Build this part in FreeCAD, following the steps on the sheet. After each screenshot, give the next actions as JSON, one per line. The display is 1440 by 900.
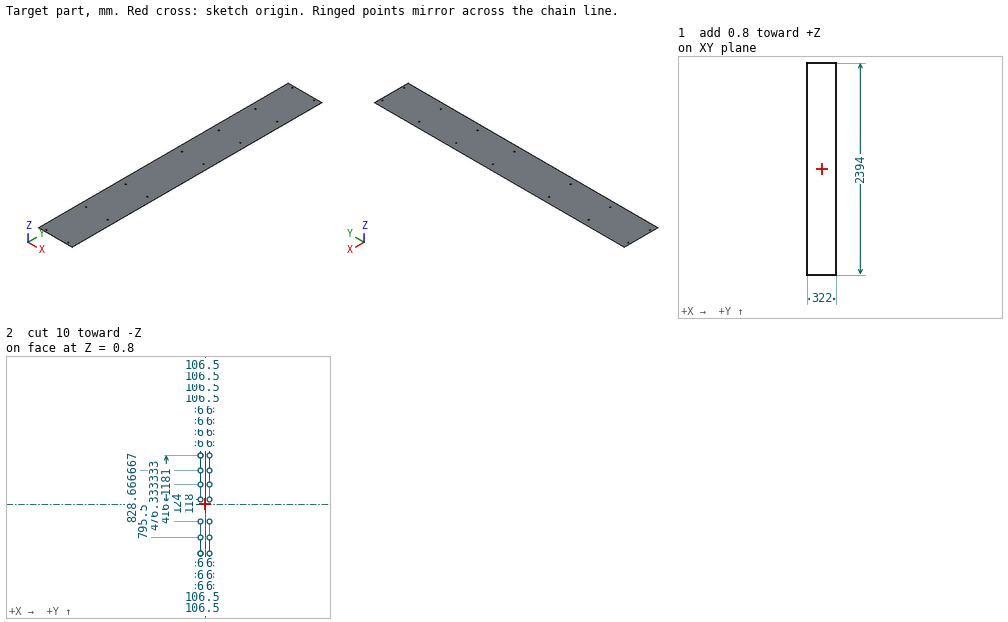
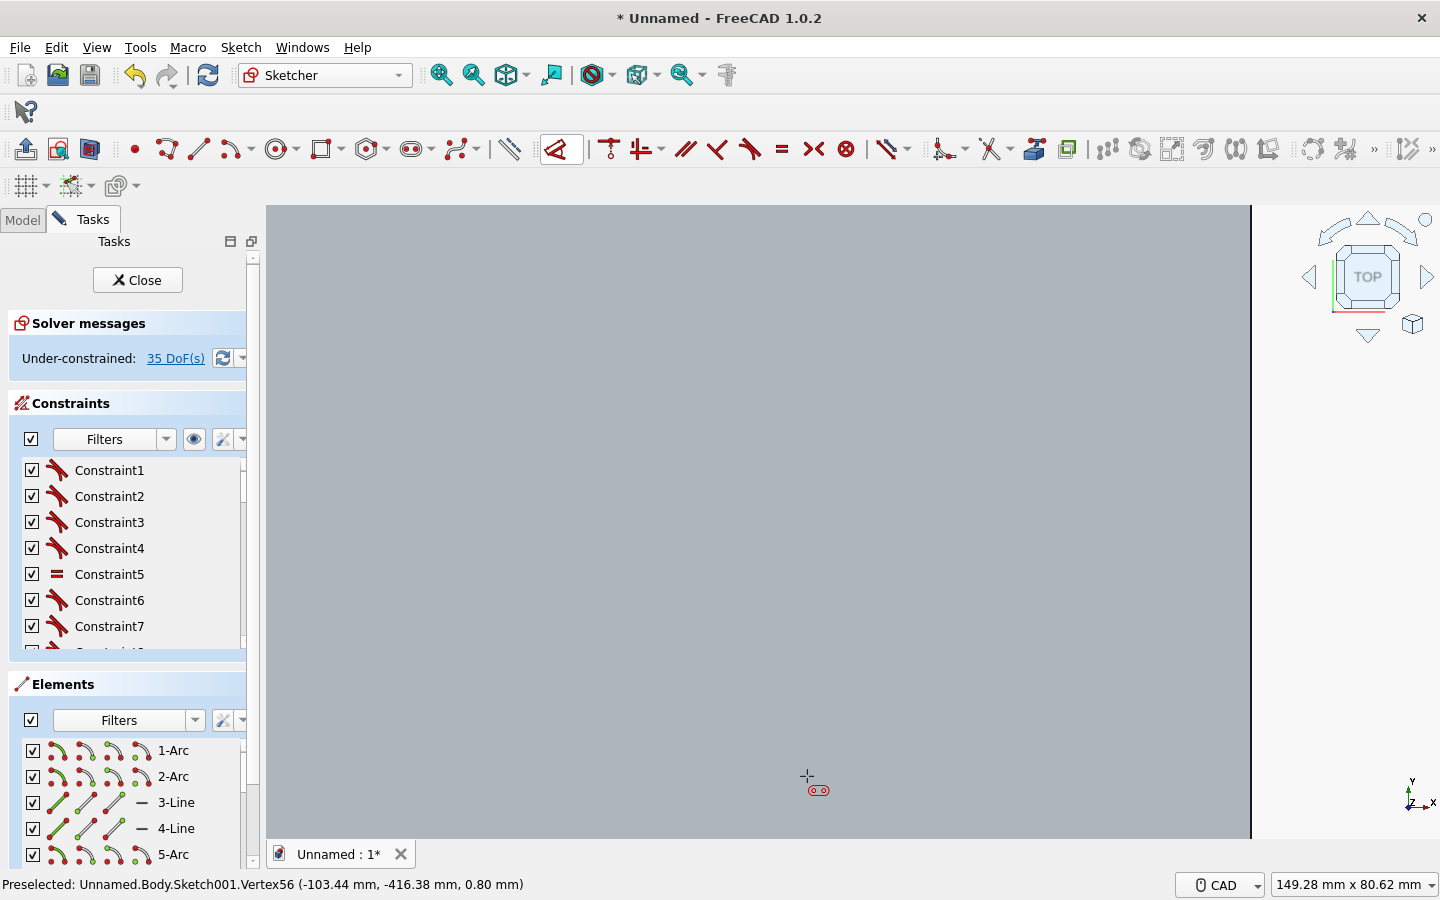
{"action": "scroll", "coordinate": [807, 776], "scroll_direction": "down", "scroll_amount": 18}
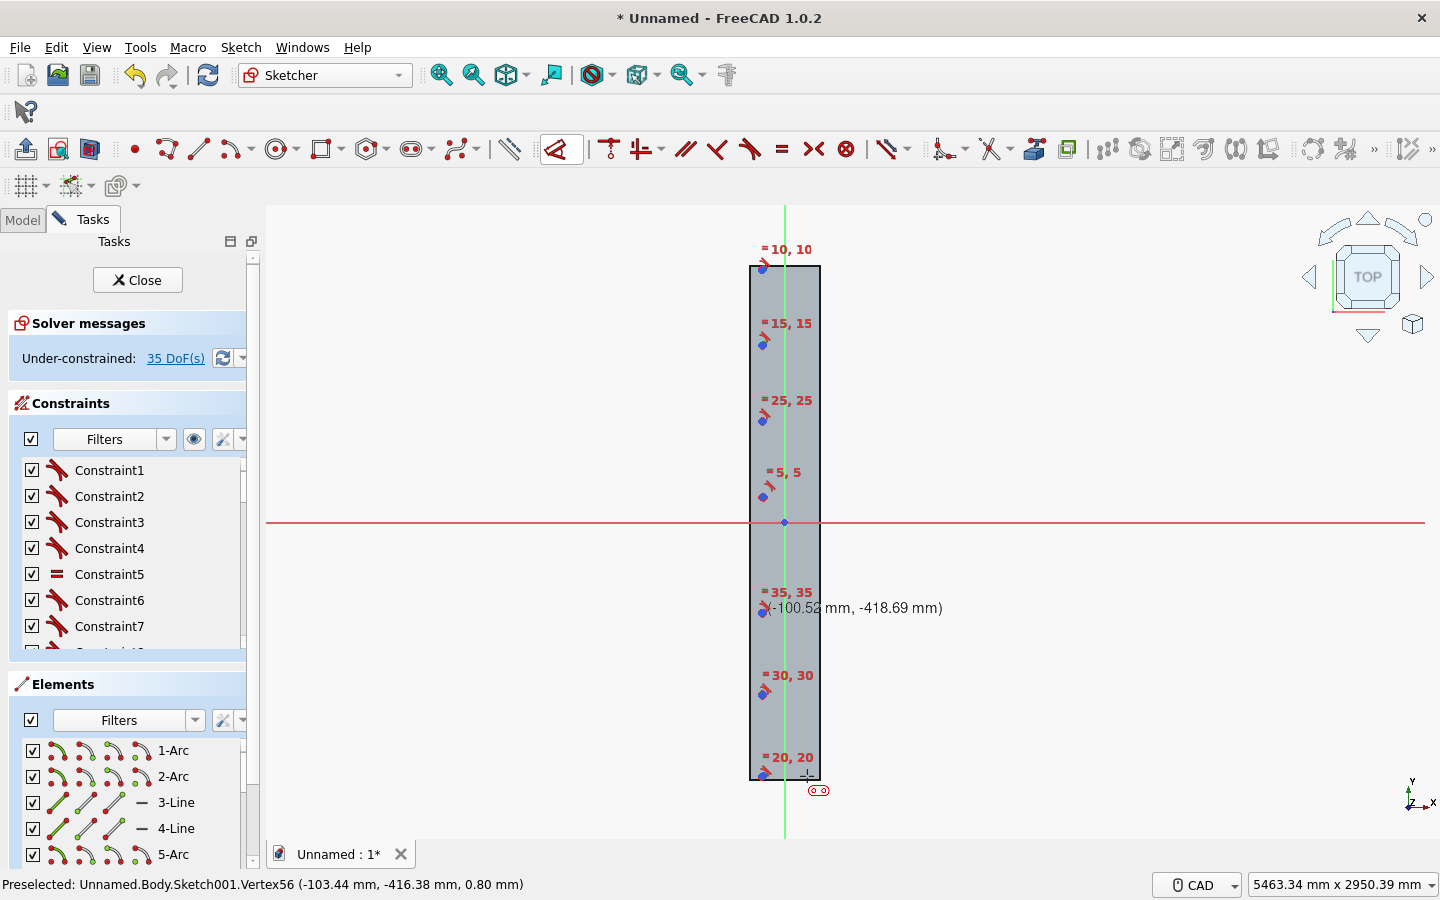
{"action": "left_click", "coordinate": [807, 776]}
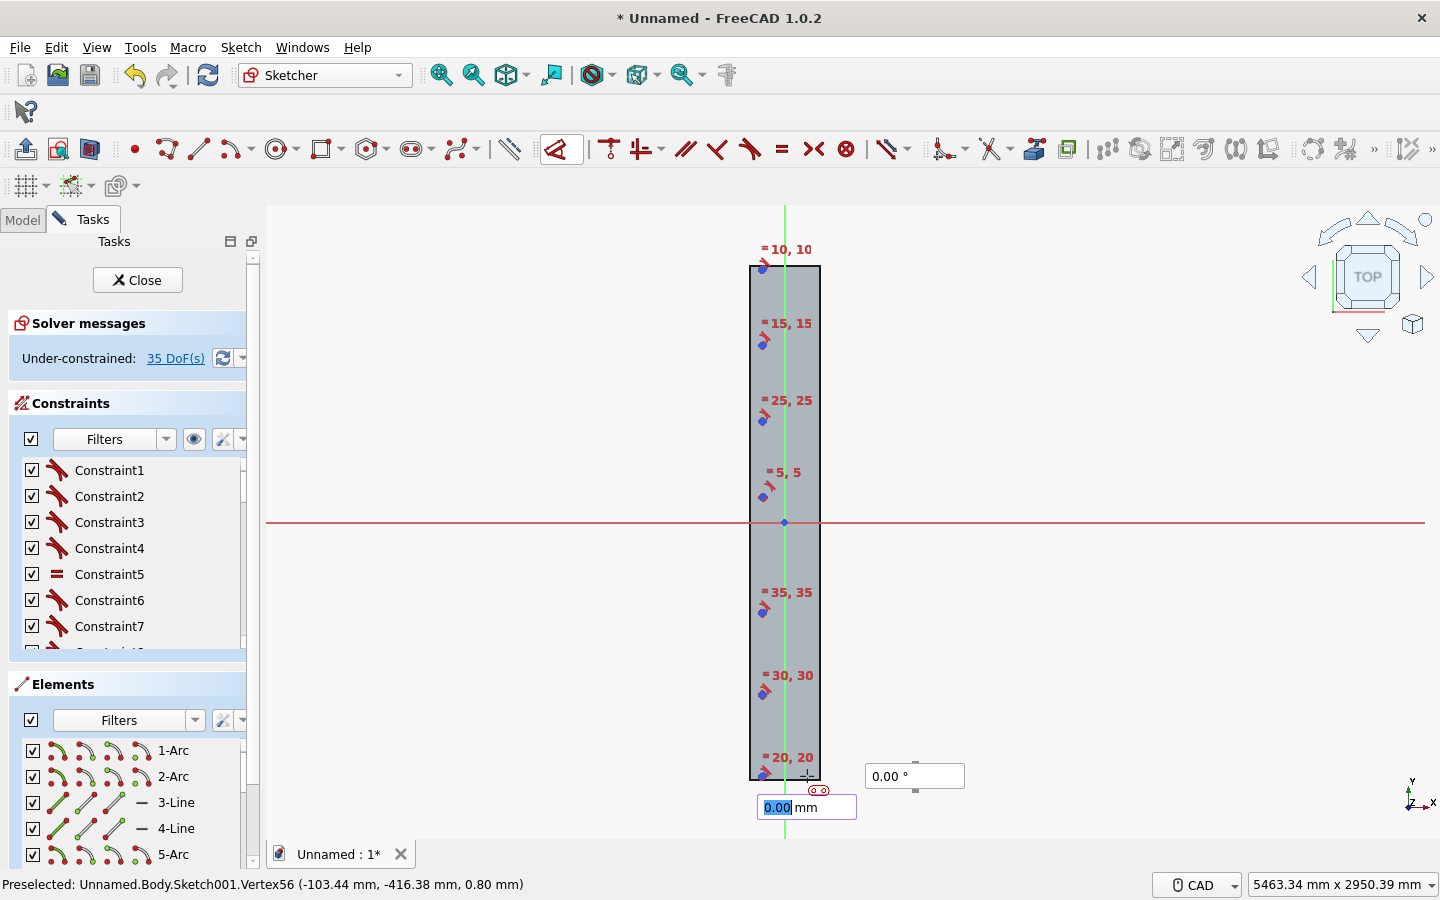
{"action": "scroll", "coordinate": [808, 776], "scroll_direction": "up", "scroll_amount": 13}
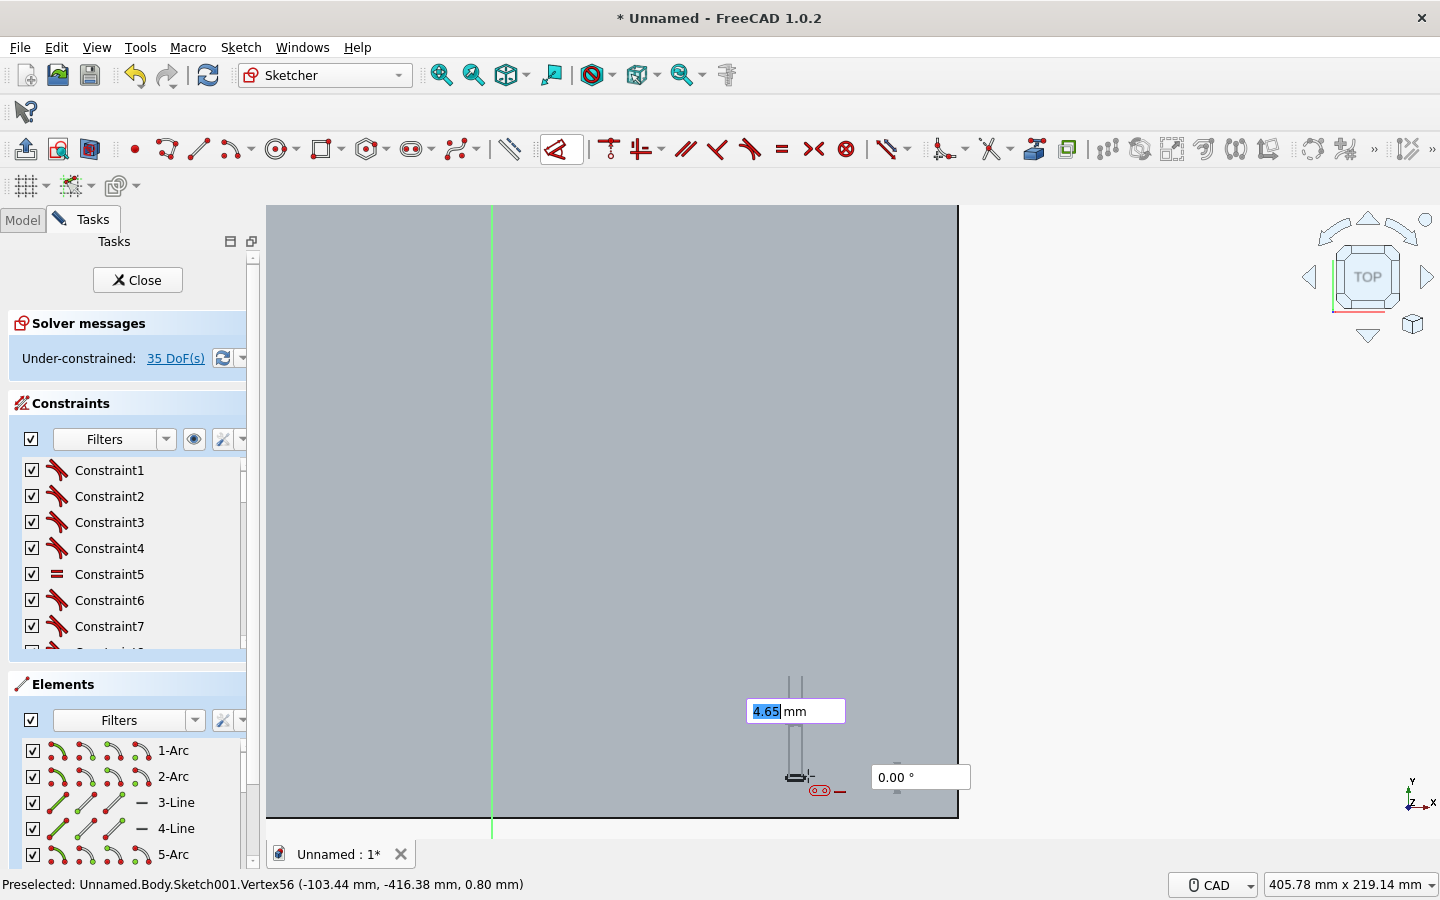
{"action": "left_click", "coordinate": [801, 765]}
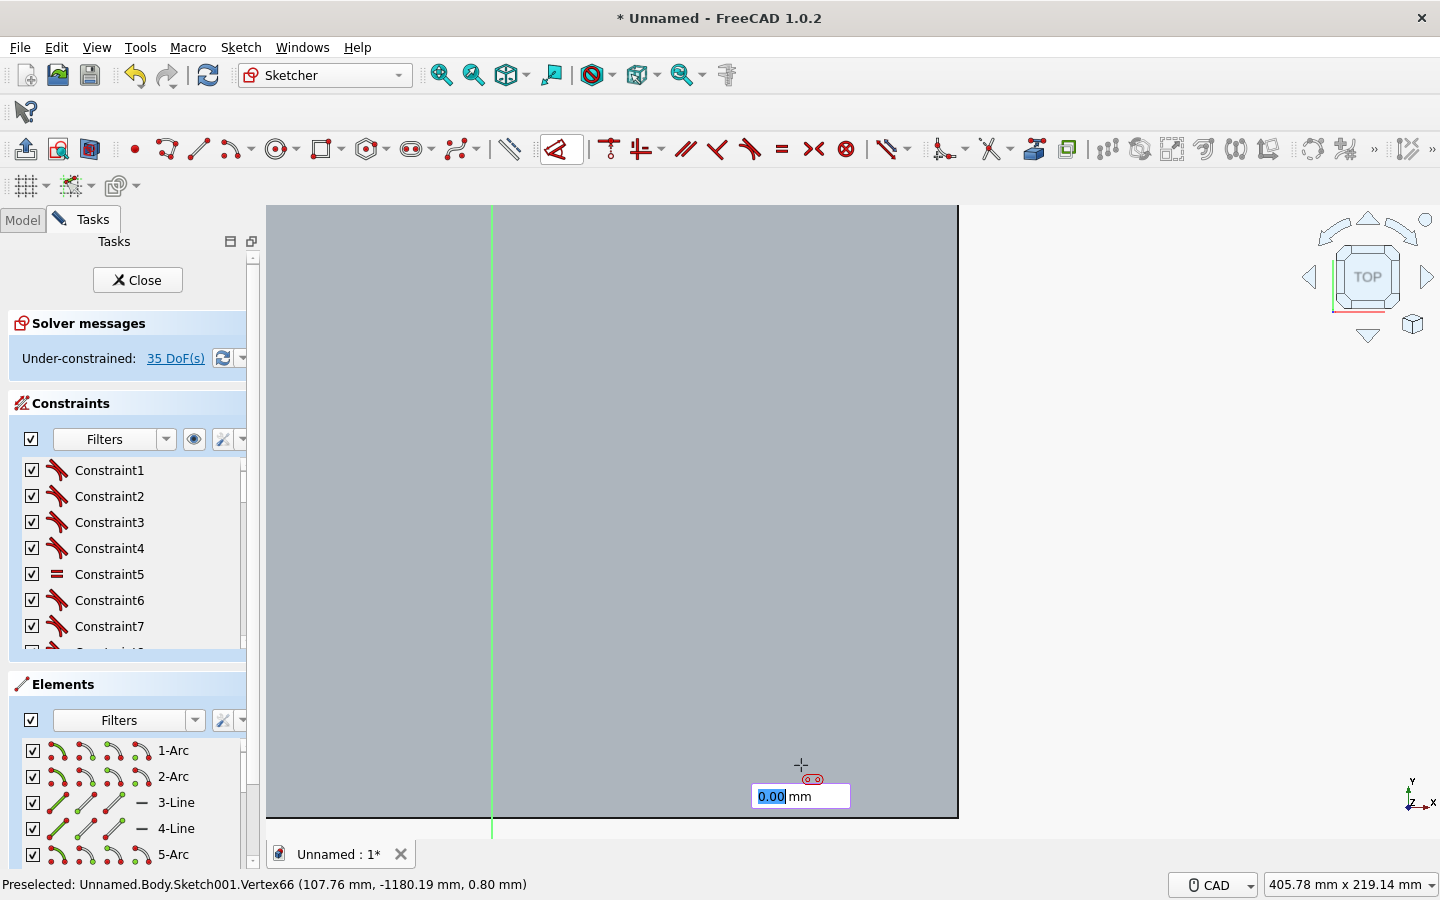
{"action": "scroll", "coordinate": [792, 755], "scroll_direction": "up", "scroll_amount": 4}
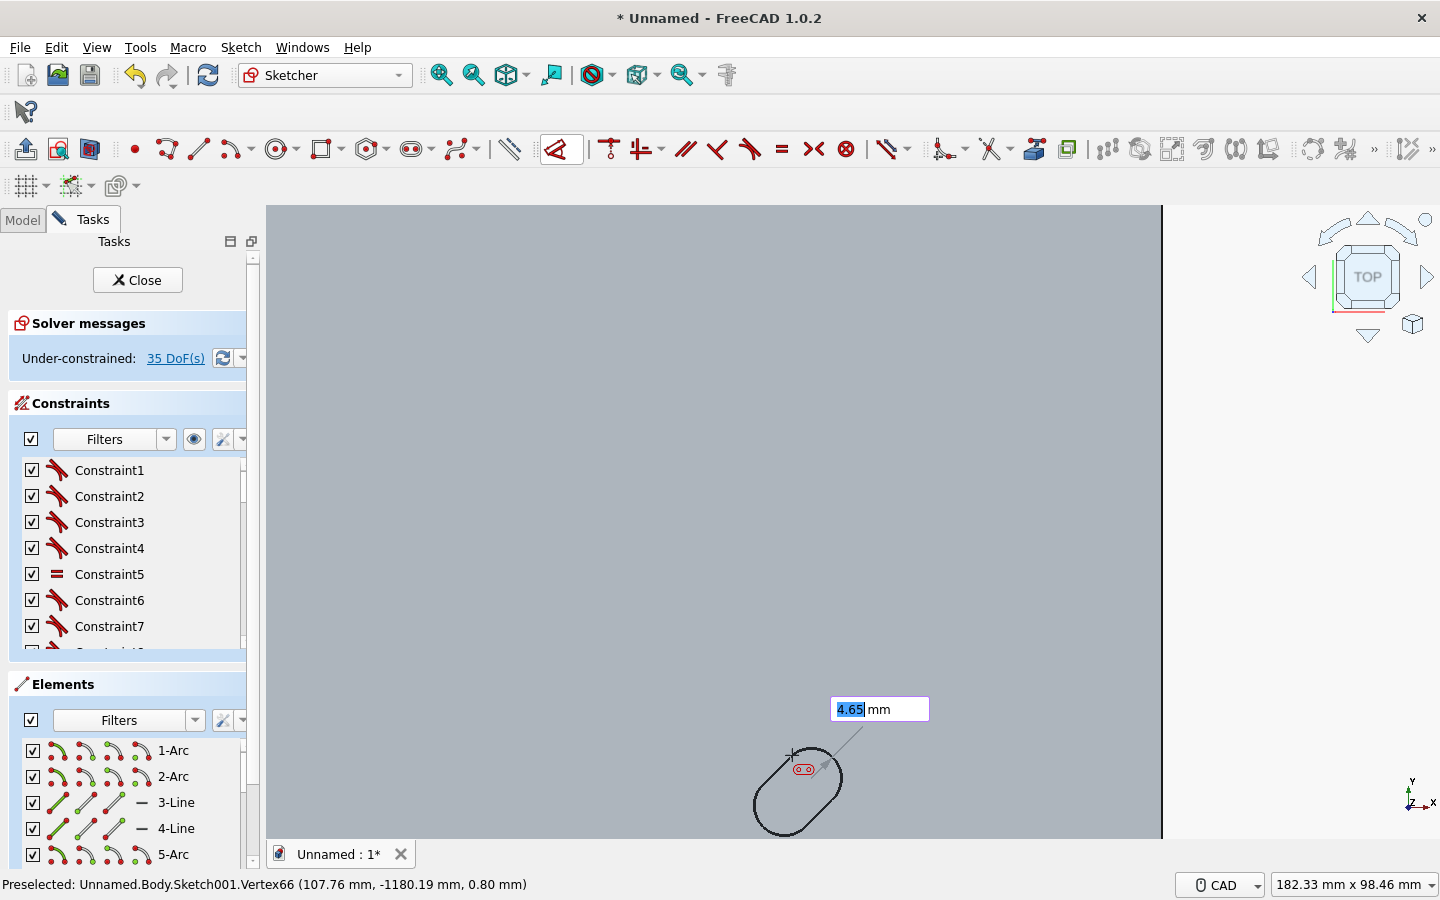
{"action": "left_click", "coordinate": [791, 753]}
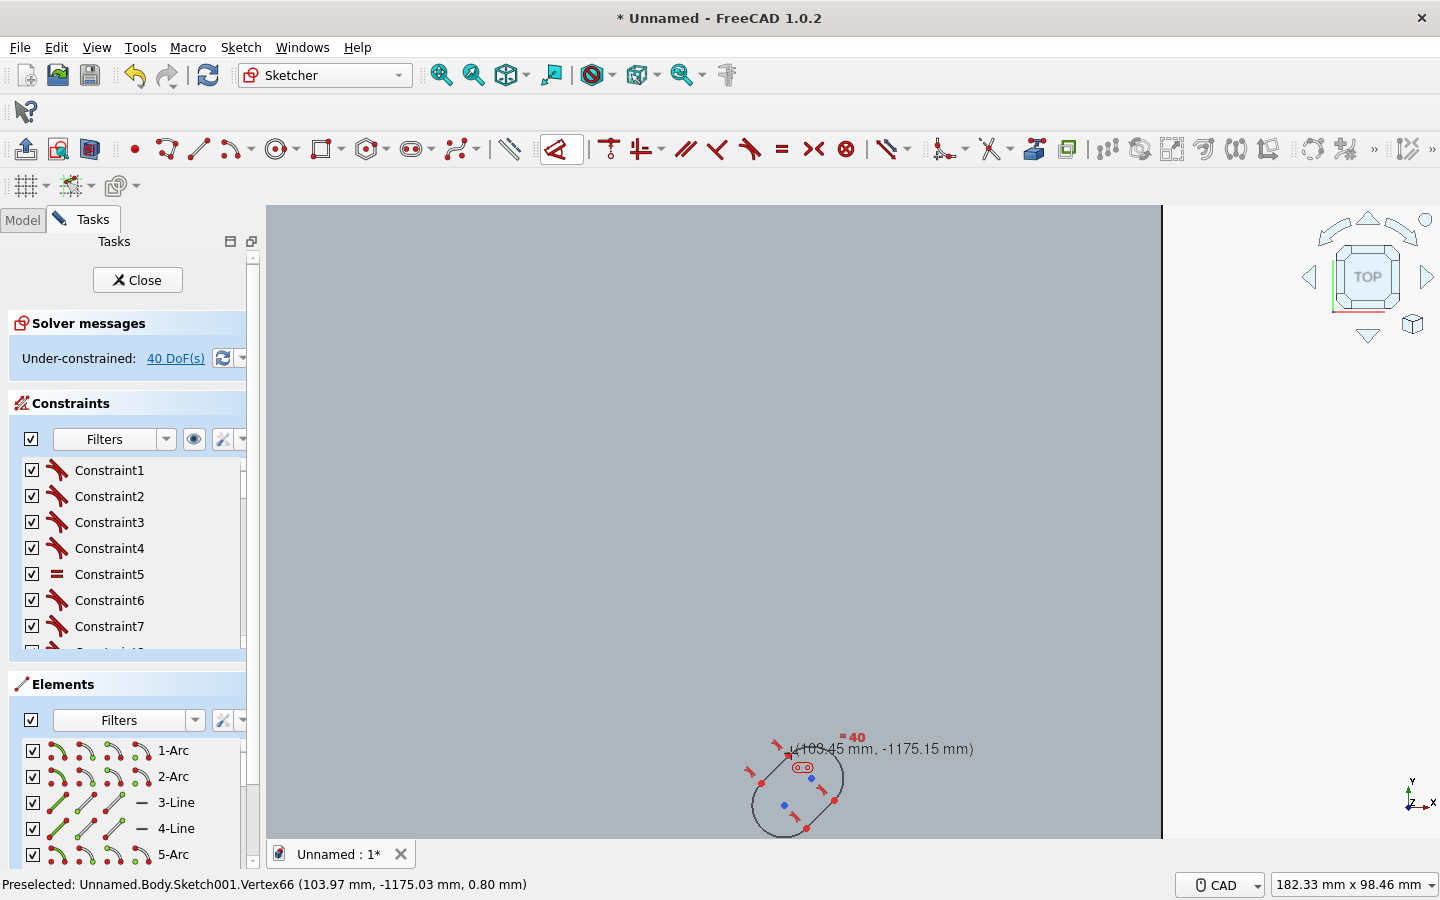
{"action": "scroll", "coordinate": [807, 775], "scroll_direction": "down", "scroll_amount": 17}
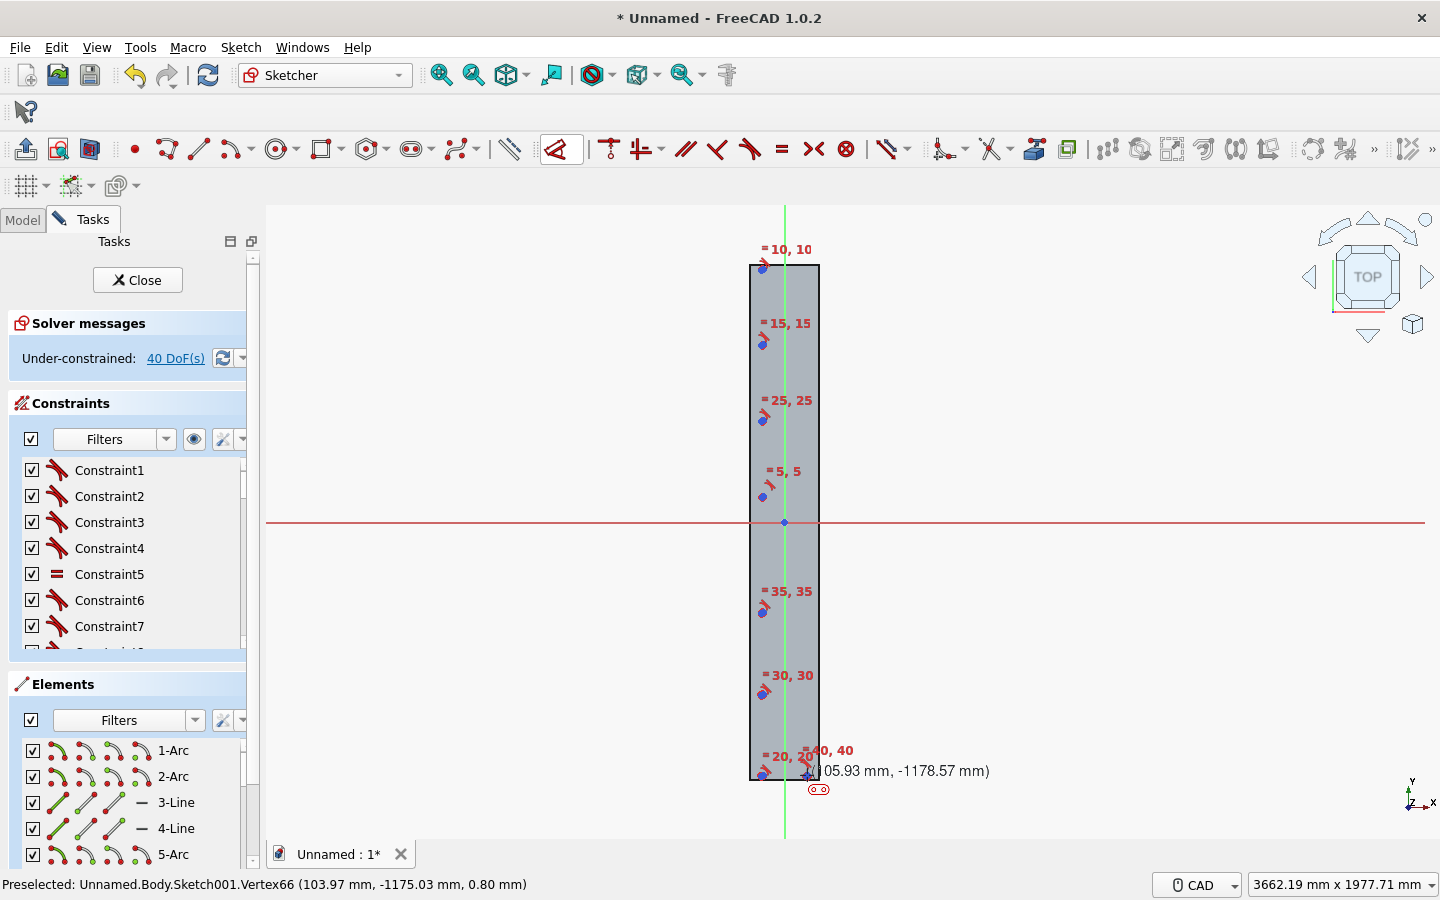
{"action": "scroll", "coordinate": [806, 694], "scroll_direction": "up", "scroll_amount": 18}